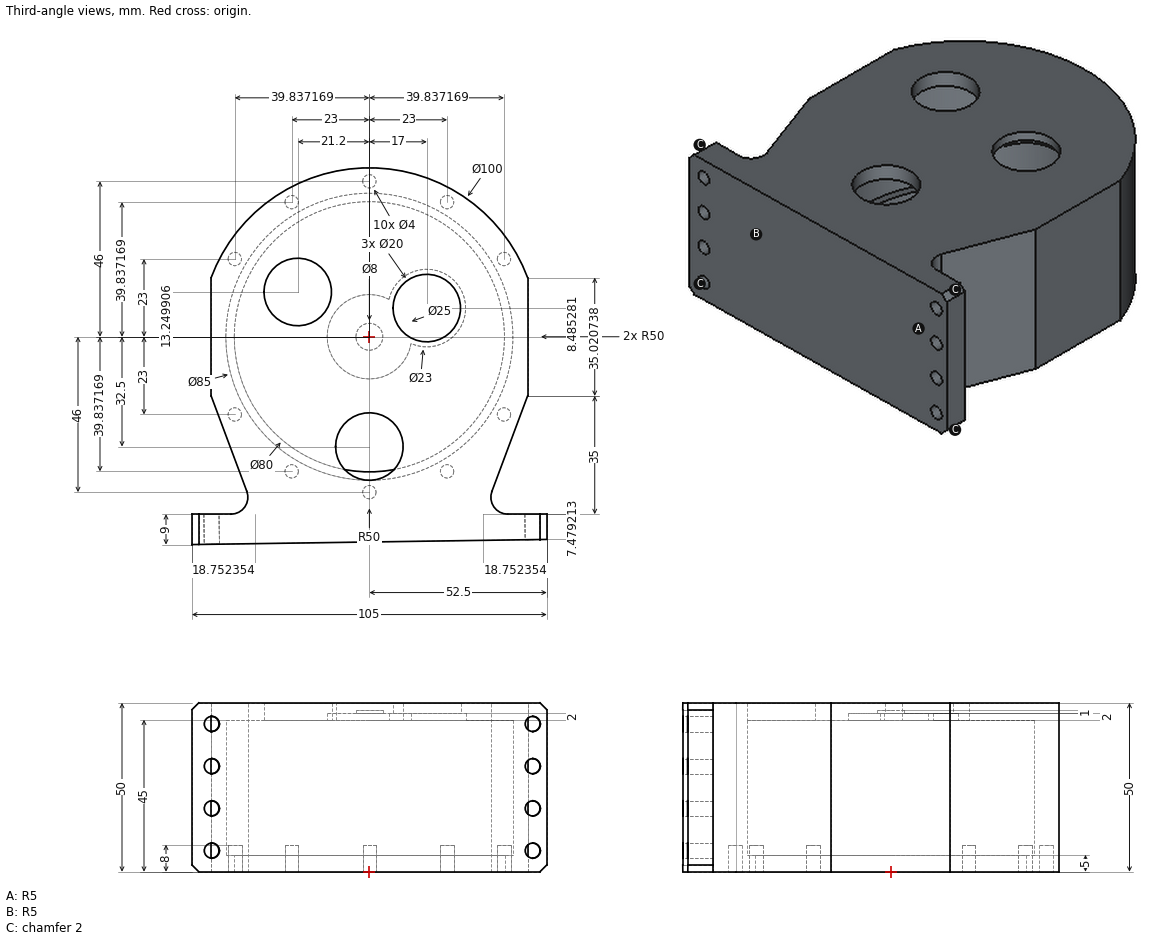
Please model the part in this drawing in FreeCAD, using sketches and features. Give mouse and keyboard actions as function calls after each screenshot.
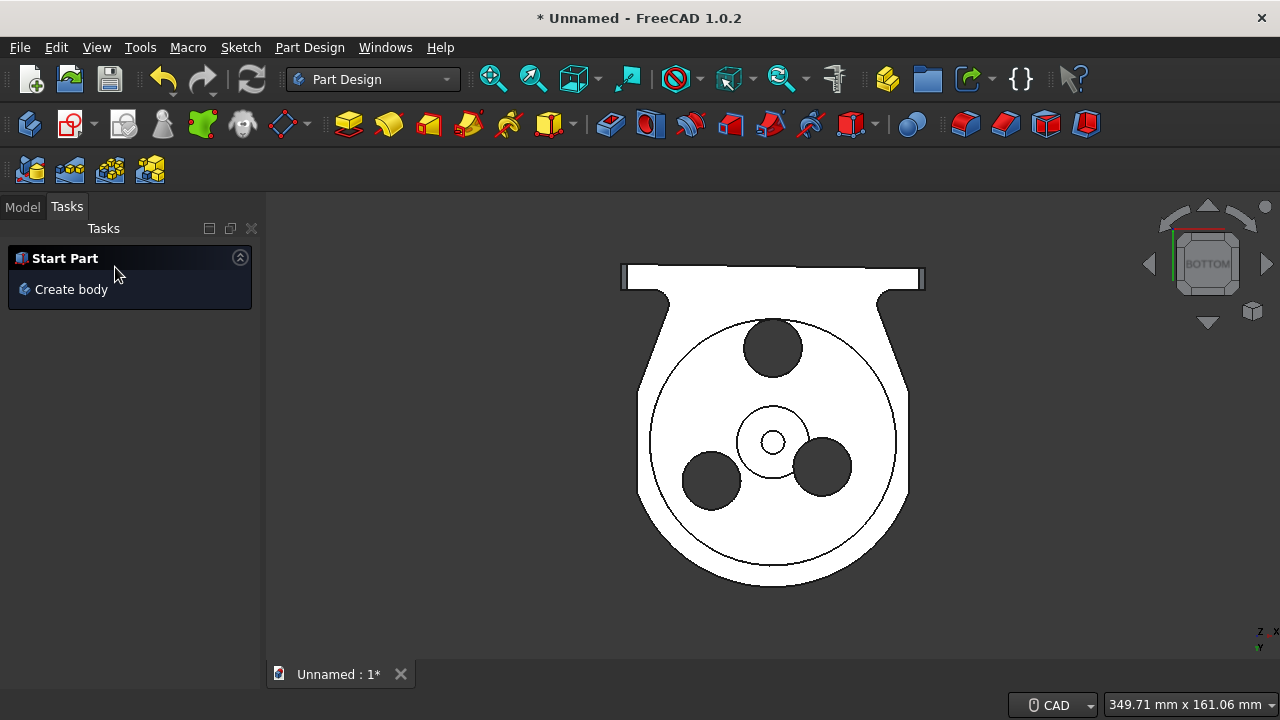
click(703, 406)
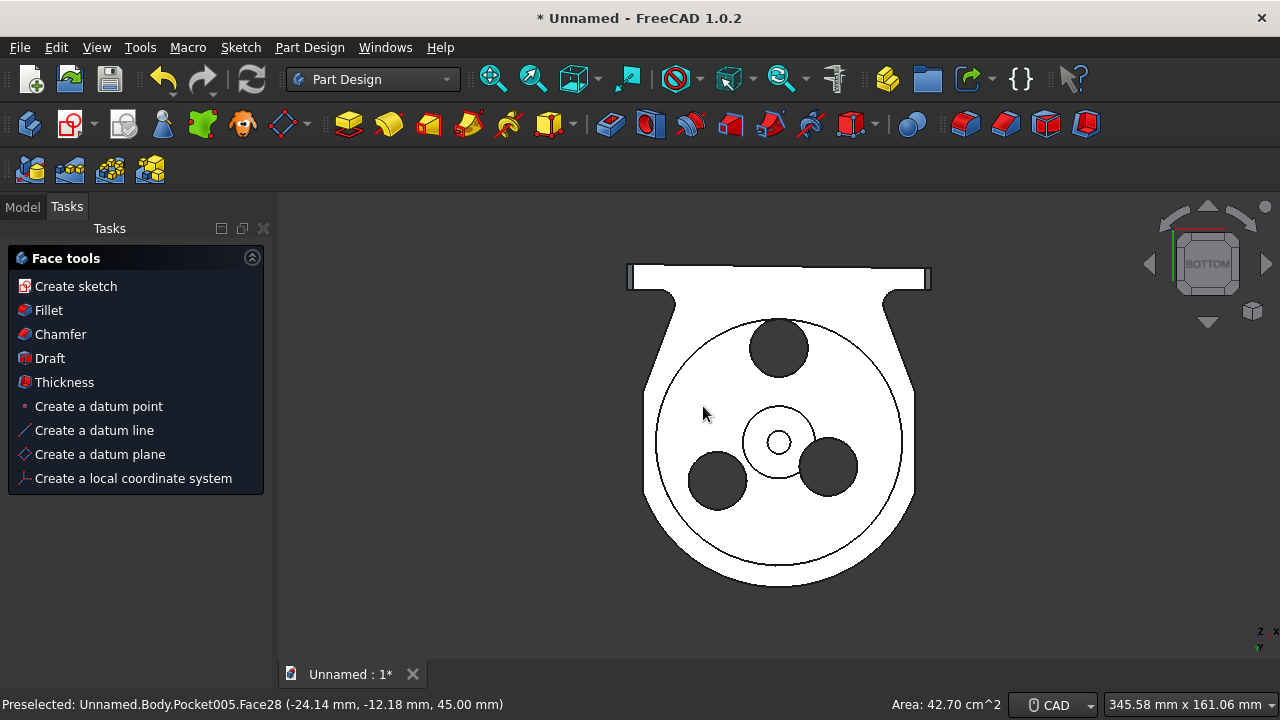
click(70, 124)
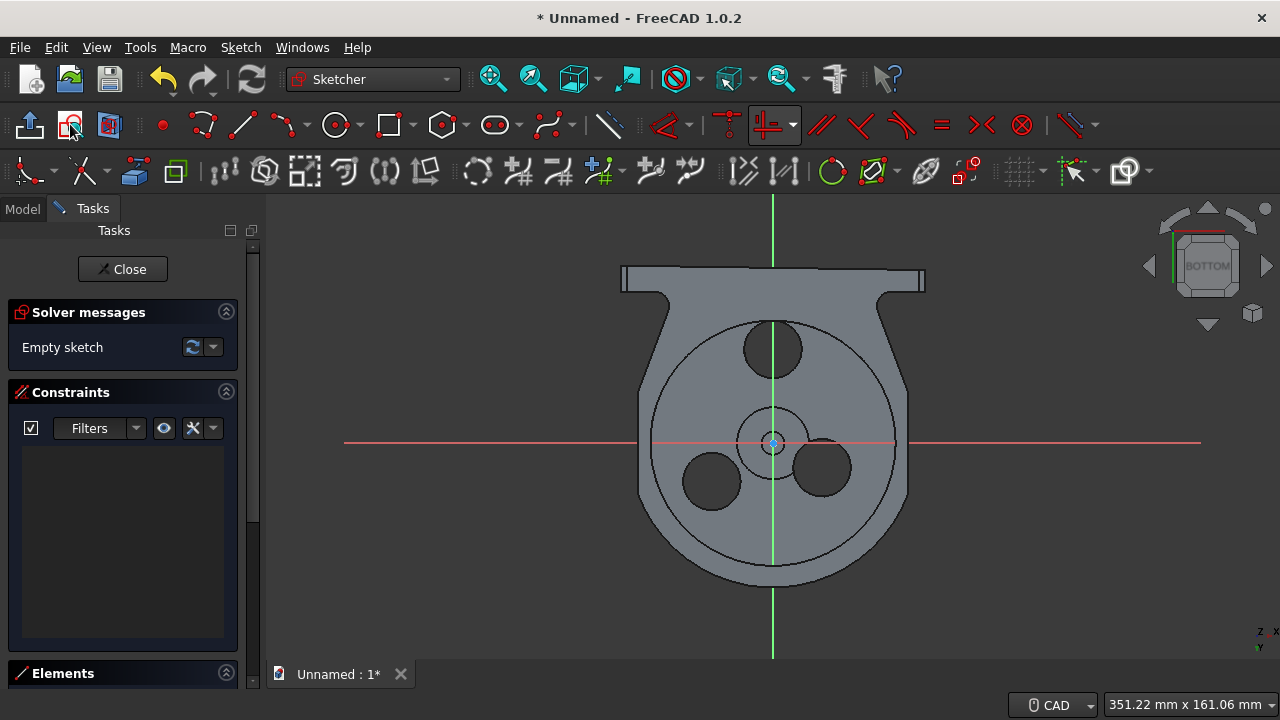
click(110, 126)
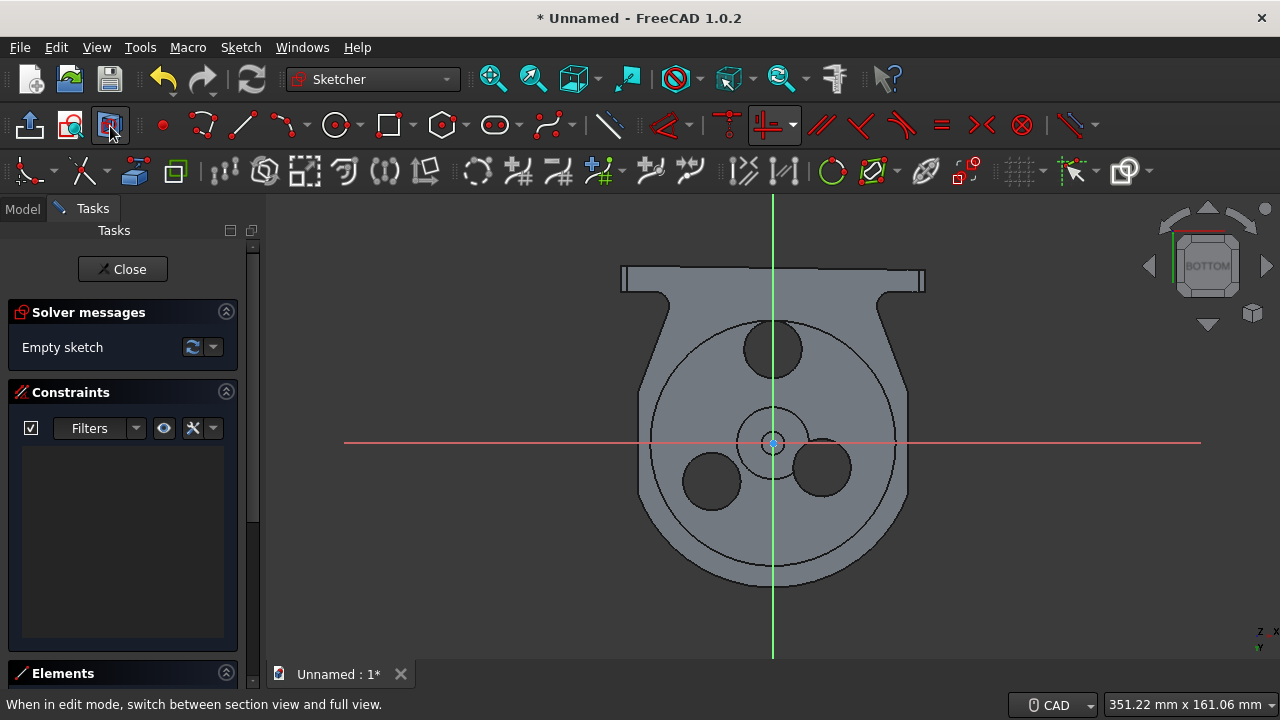
scroll(850, 481, up, 7)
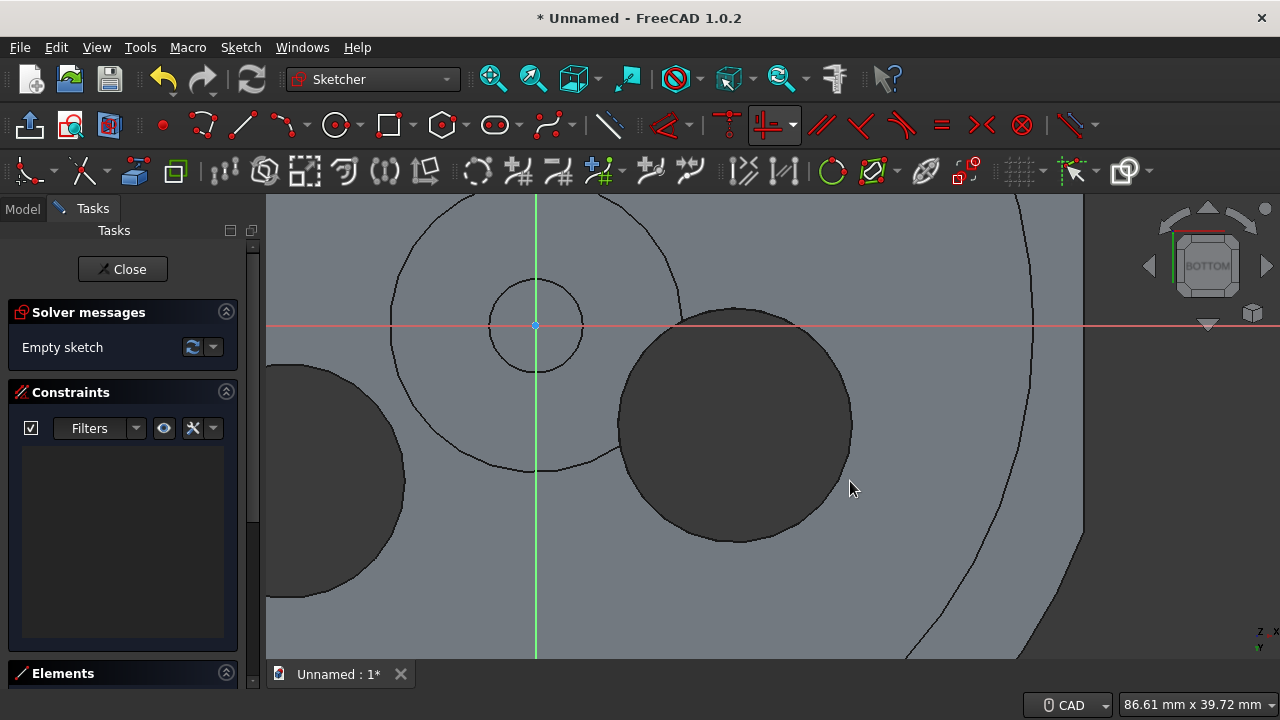
click(336, 126)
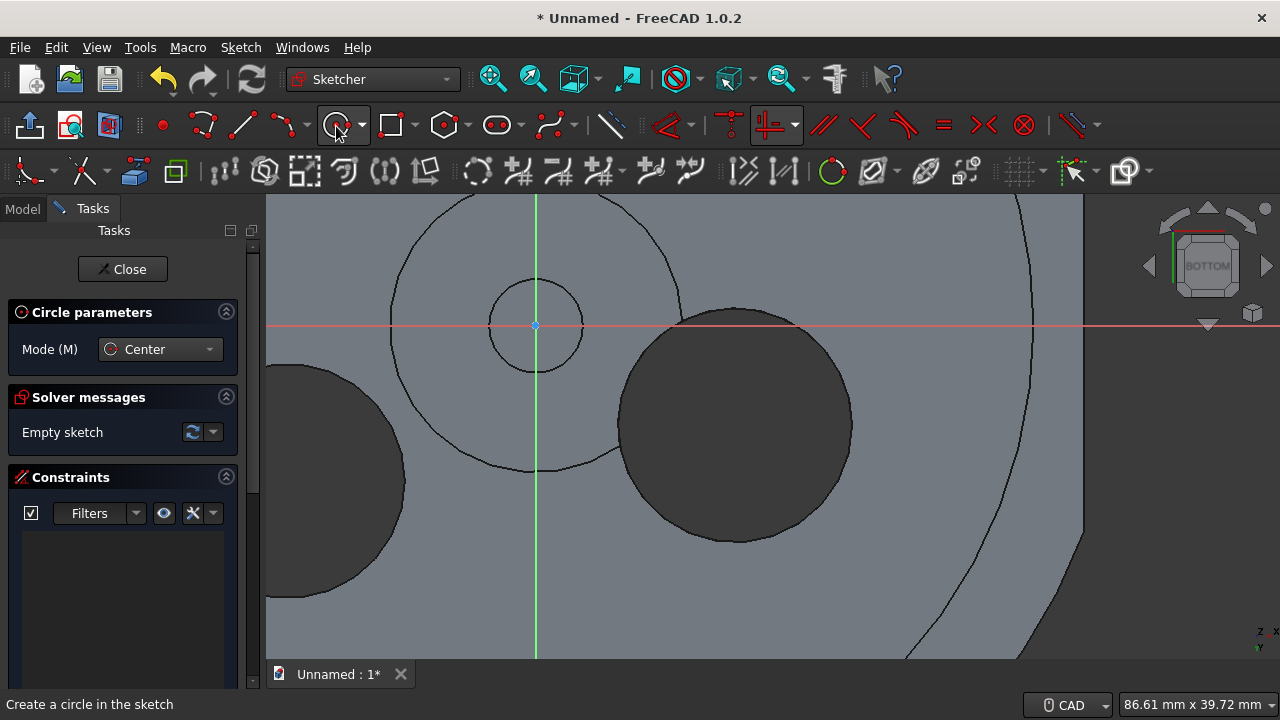
click(735, 425)
click(830, 521)
key(Escape)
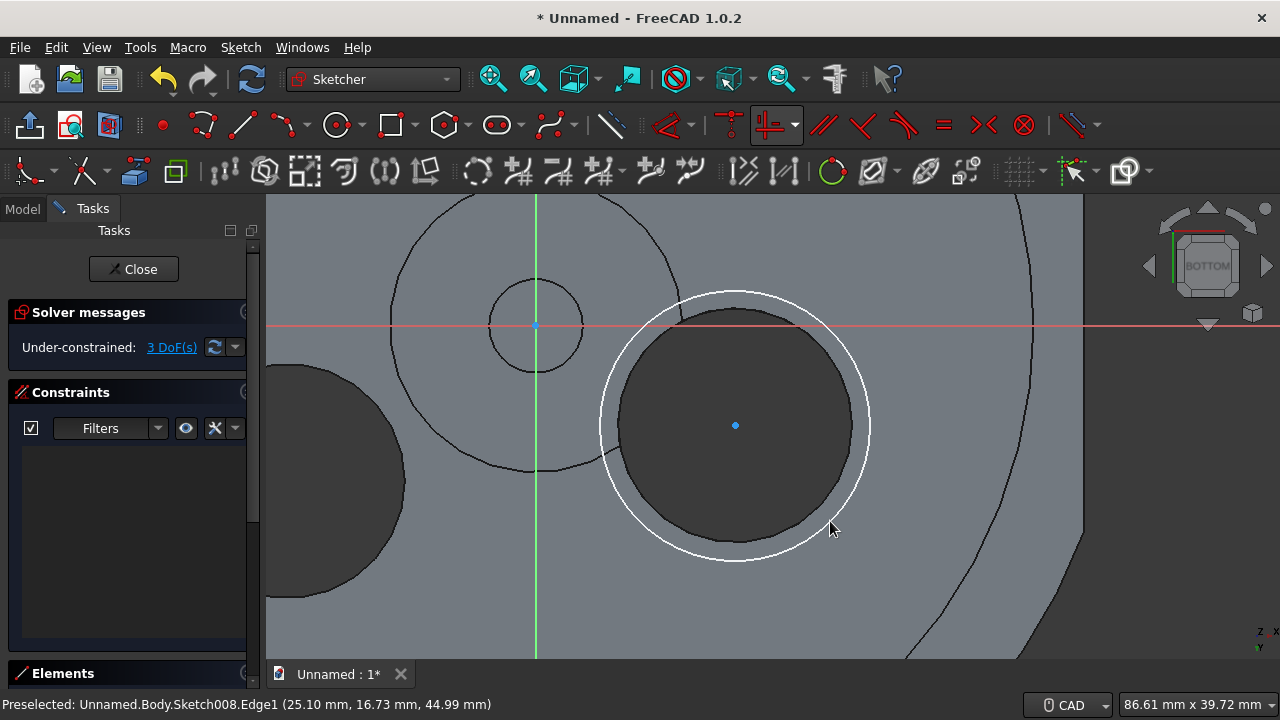
click(666, 126)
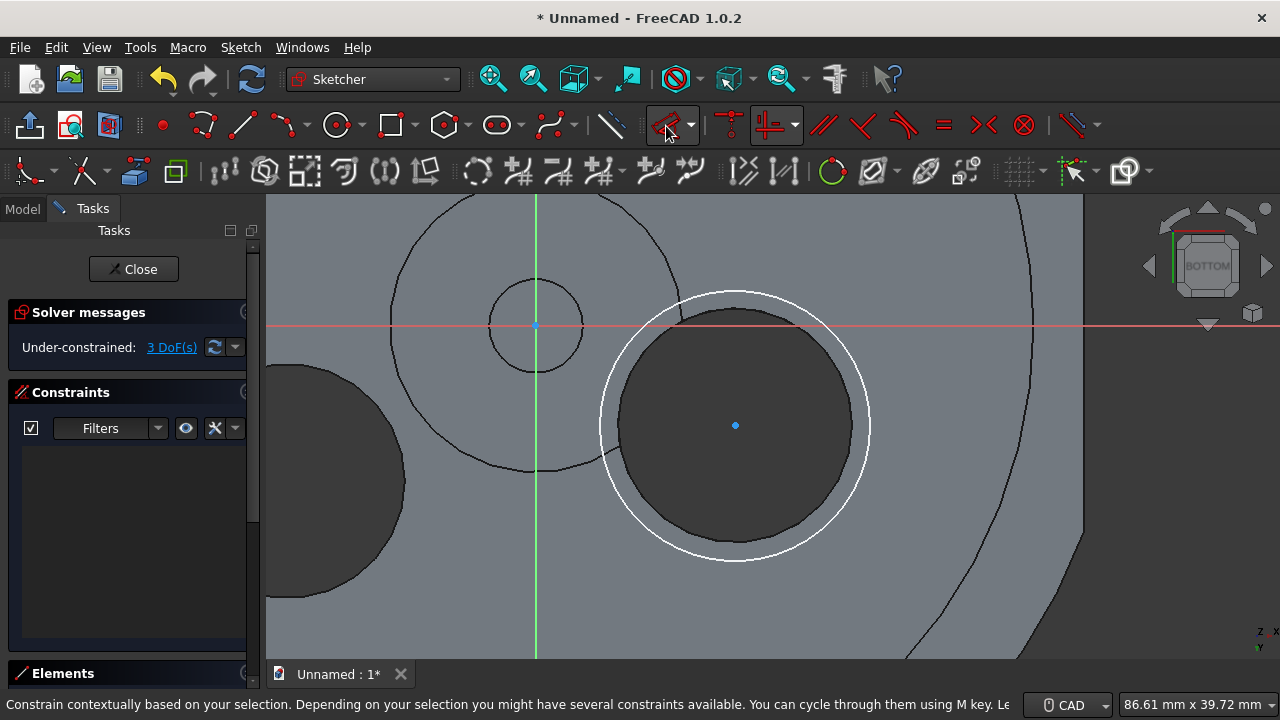
click(640, 522)
click(617, 545)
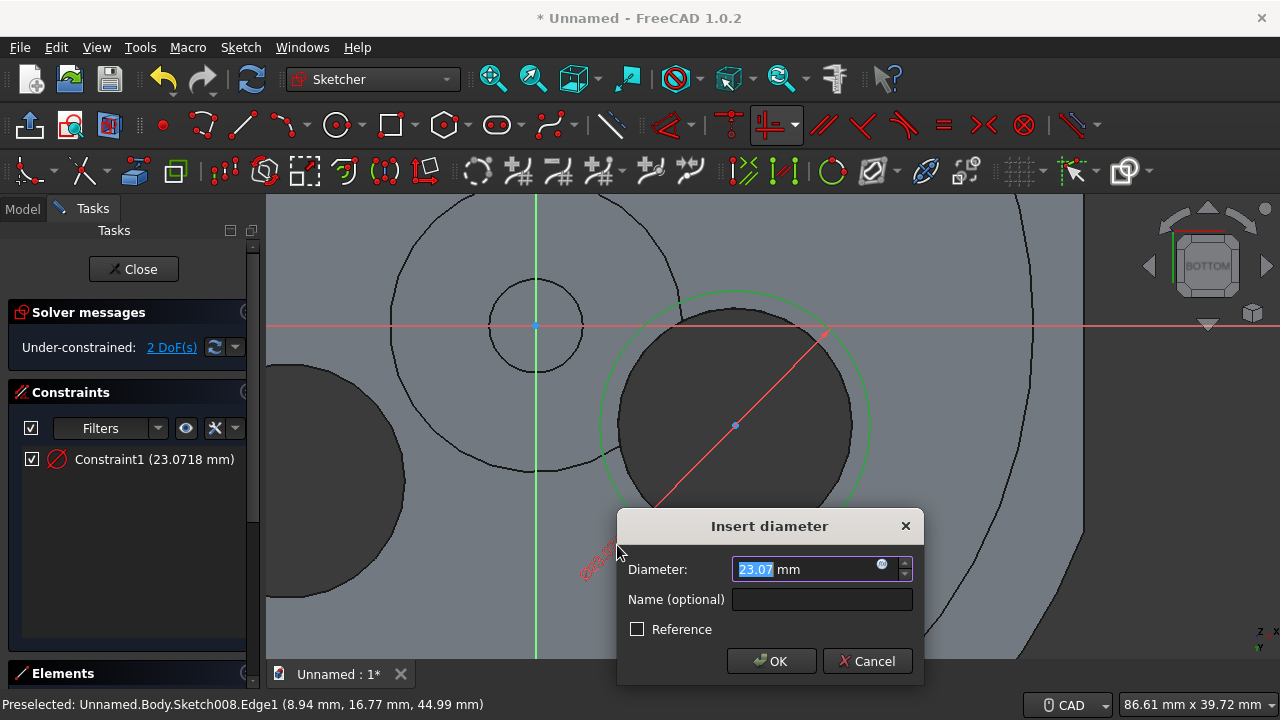
text(23)
key(Return)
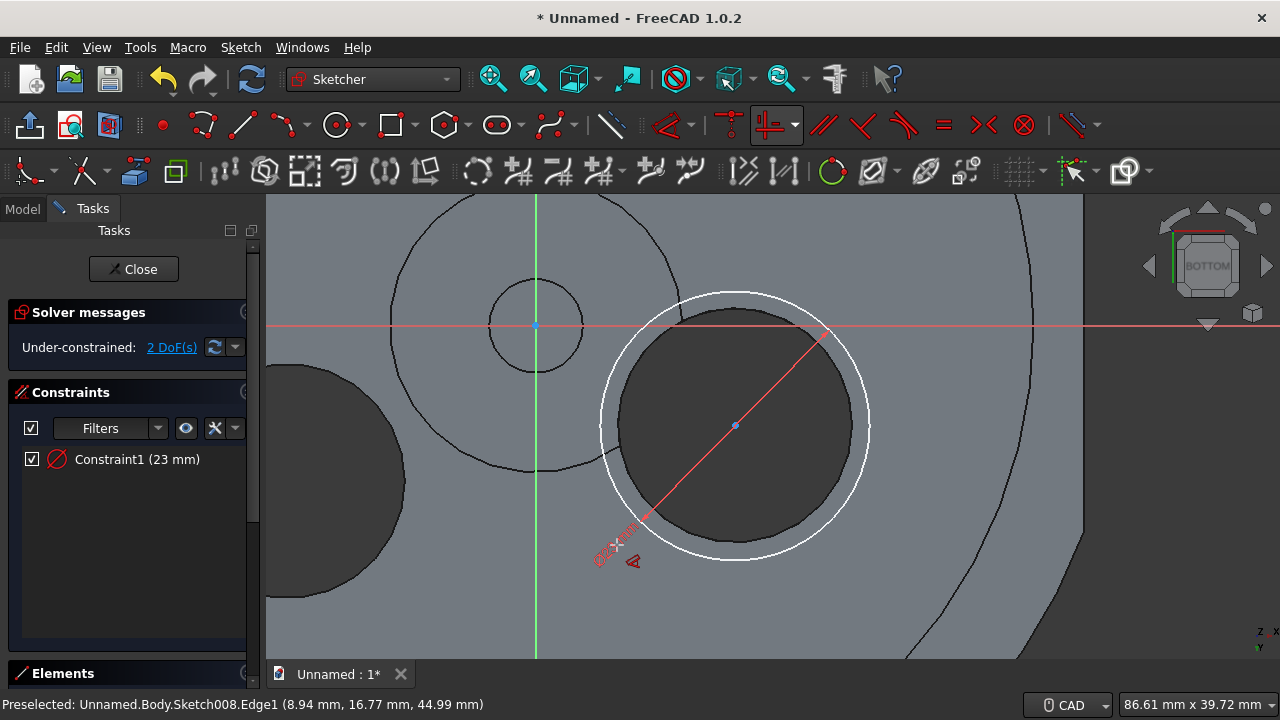
click(735, 426)
click(635, 292)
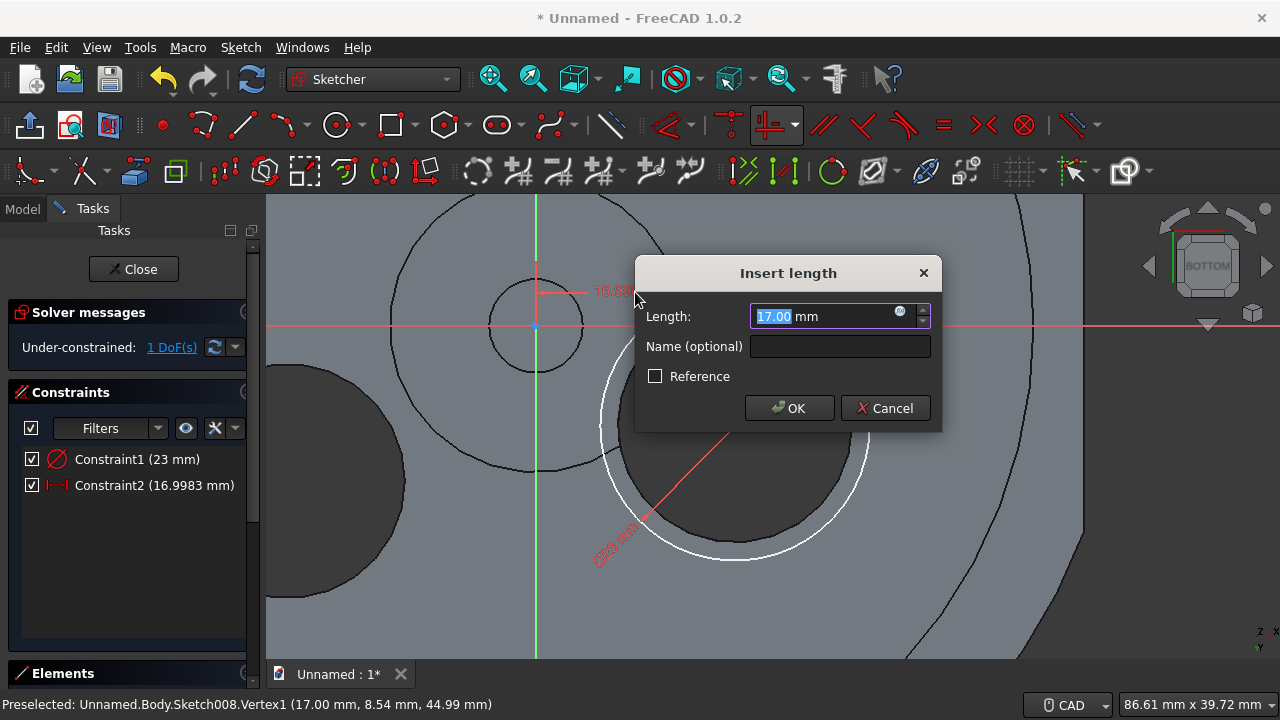
text(17)
key(Return)